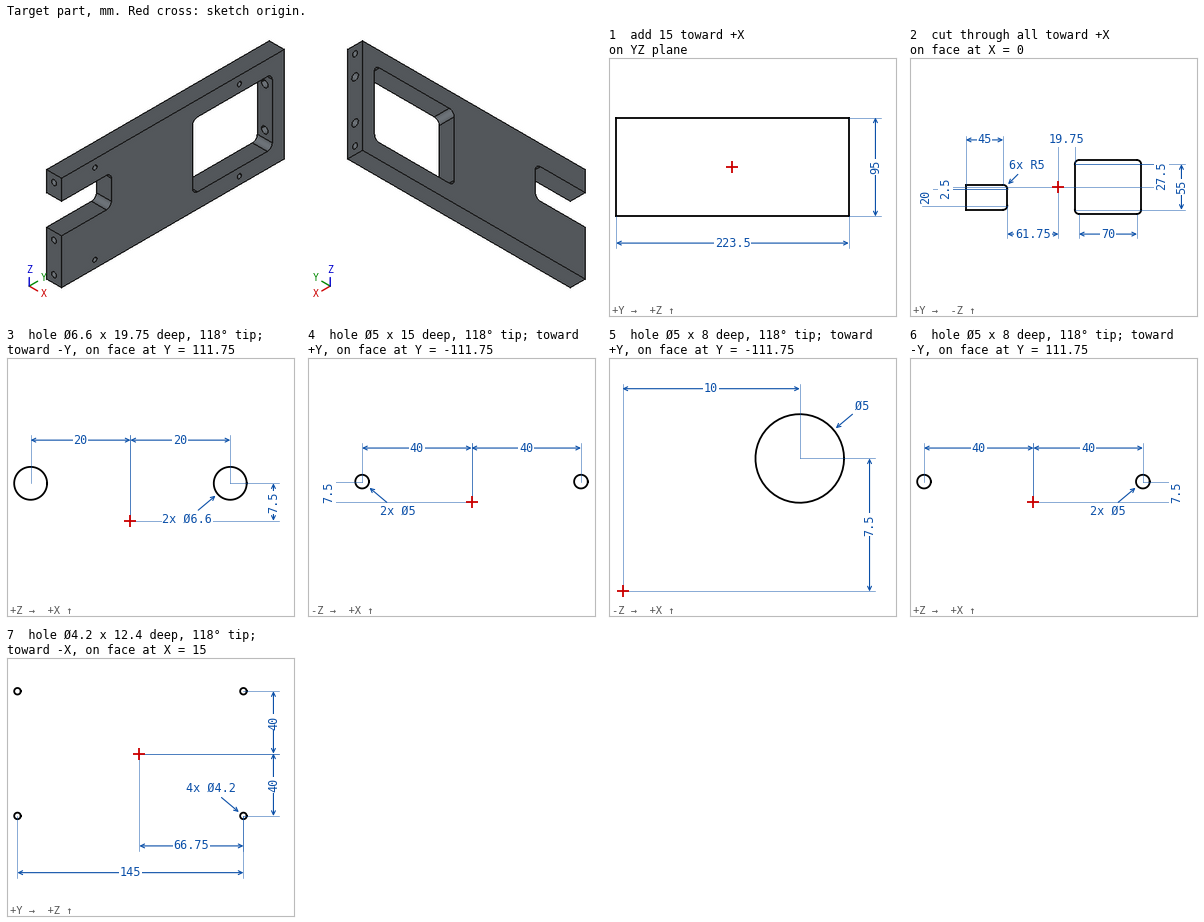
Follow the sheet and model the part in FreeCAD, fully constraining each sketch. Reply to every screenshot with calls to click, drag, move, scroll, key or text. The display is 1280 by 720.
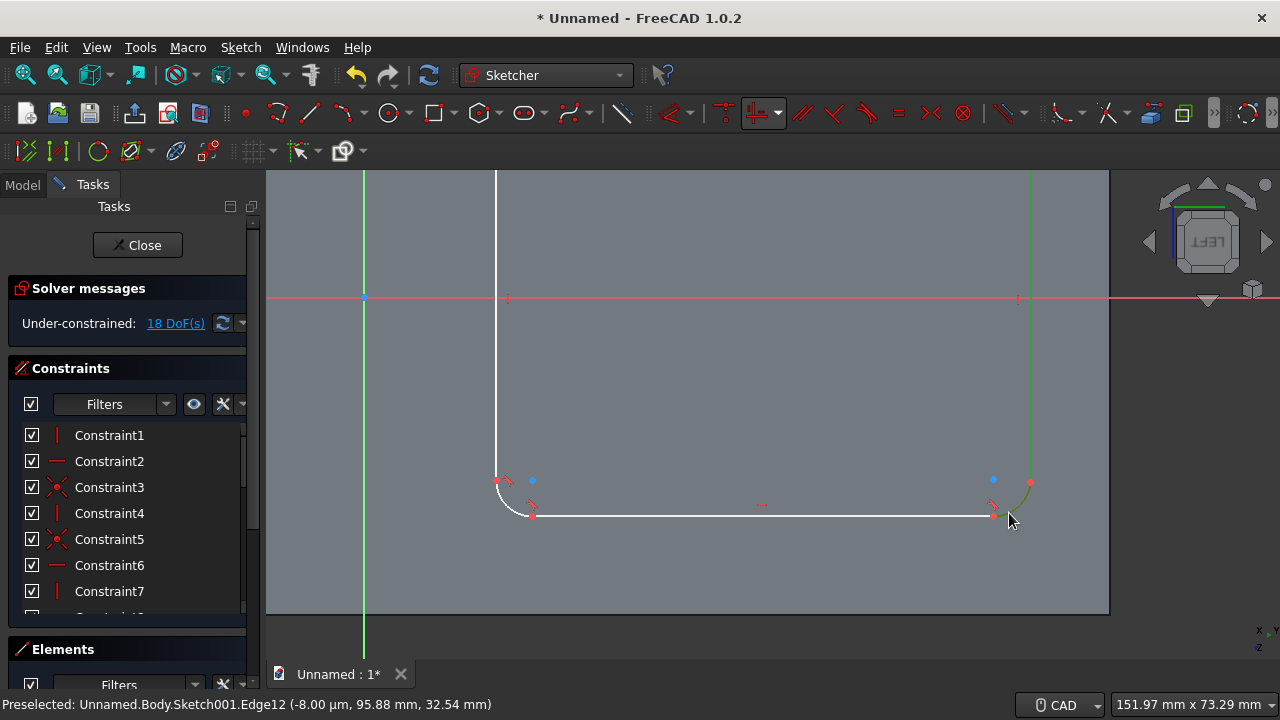
click(868, 114)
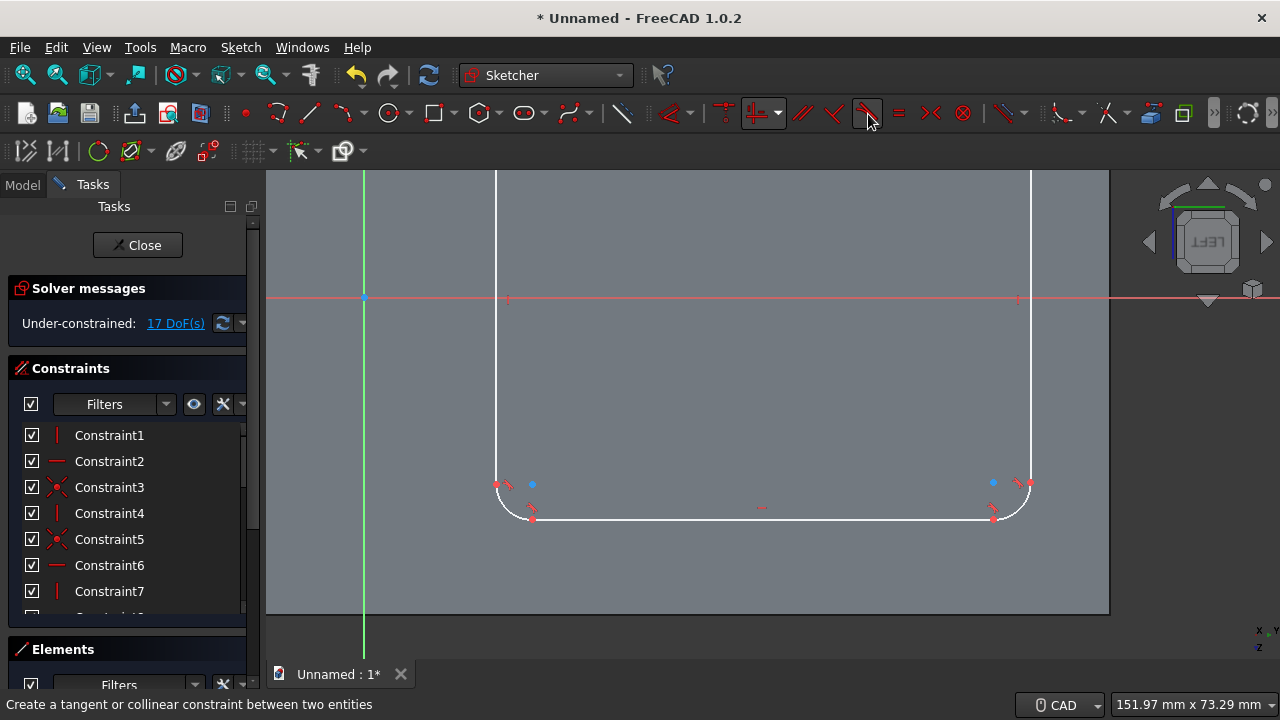
click(1031, 373)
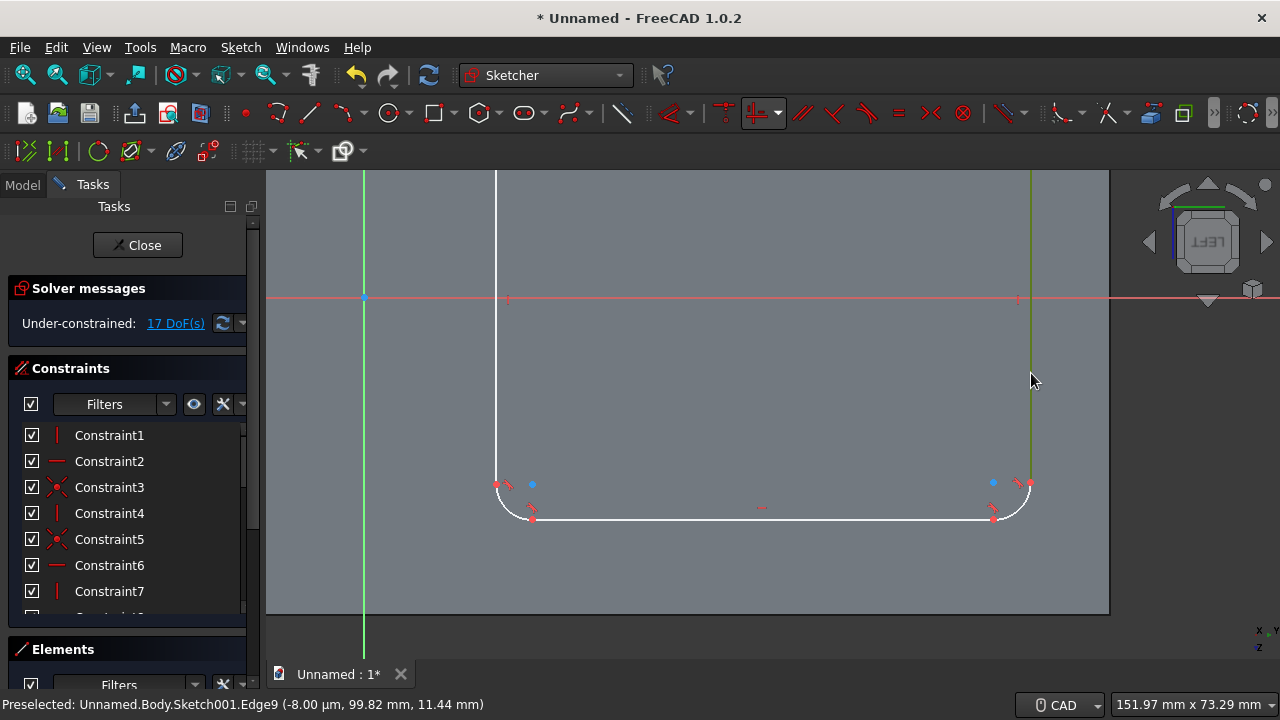
scroll(1015, 510, down, 4)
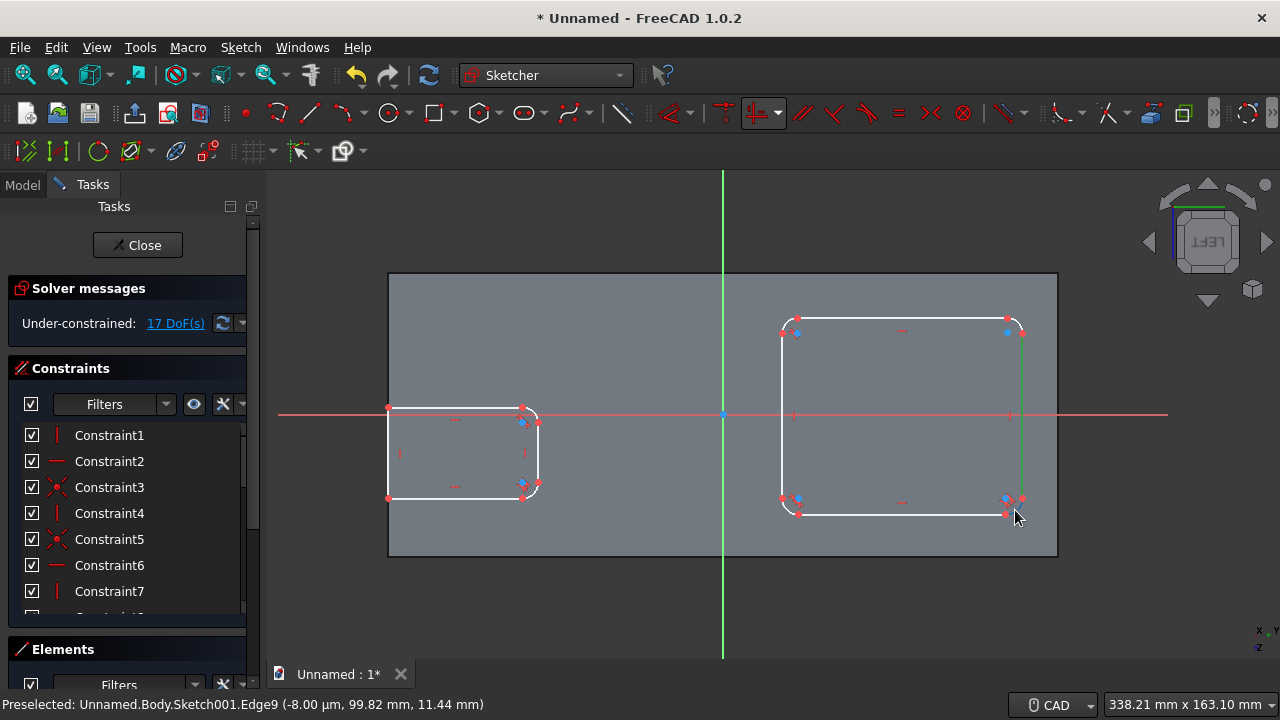
scroll(1021, 326, up, 4)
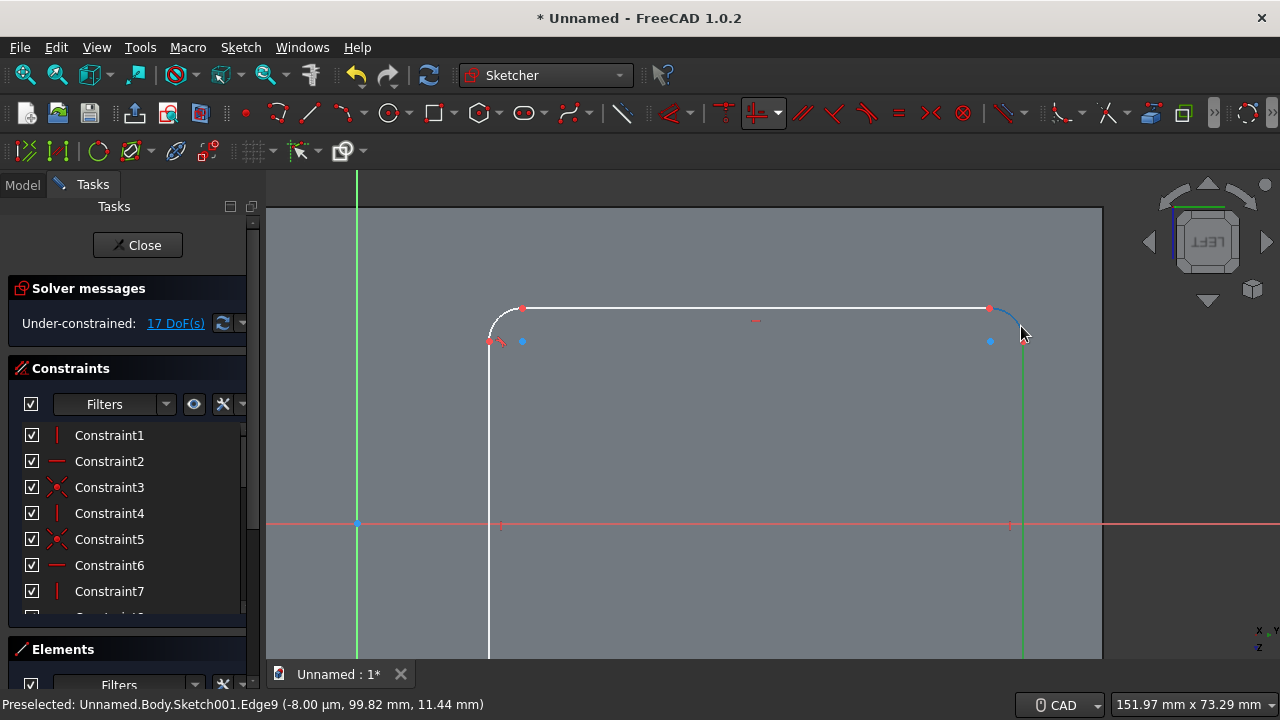
click(1020, 326)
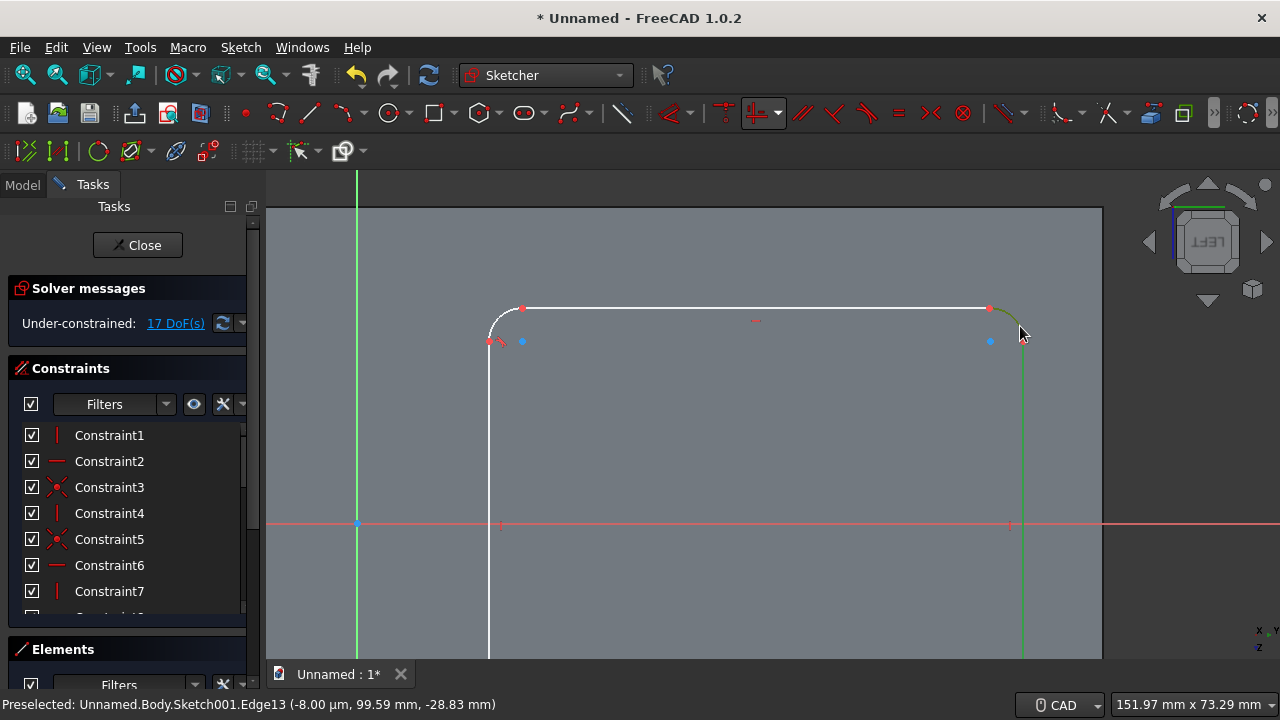
click(868, 114)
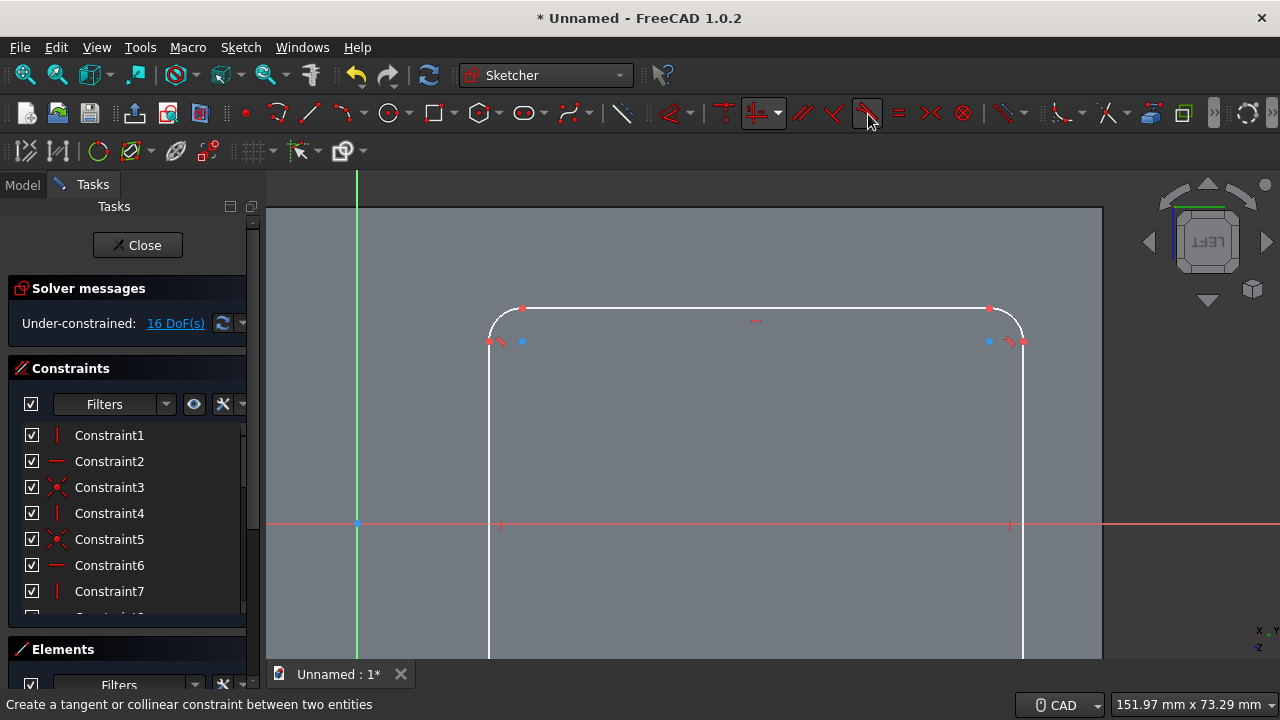
click(850, 308)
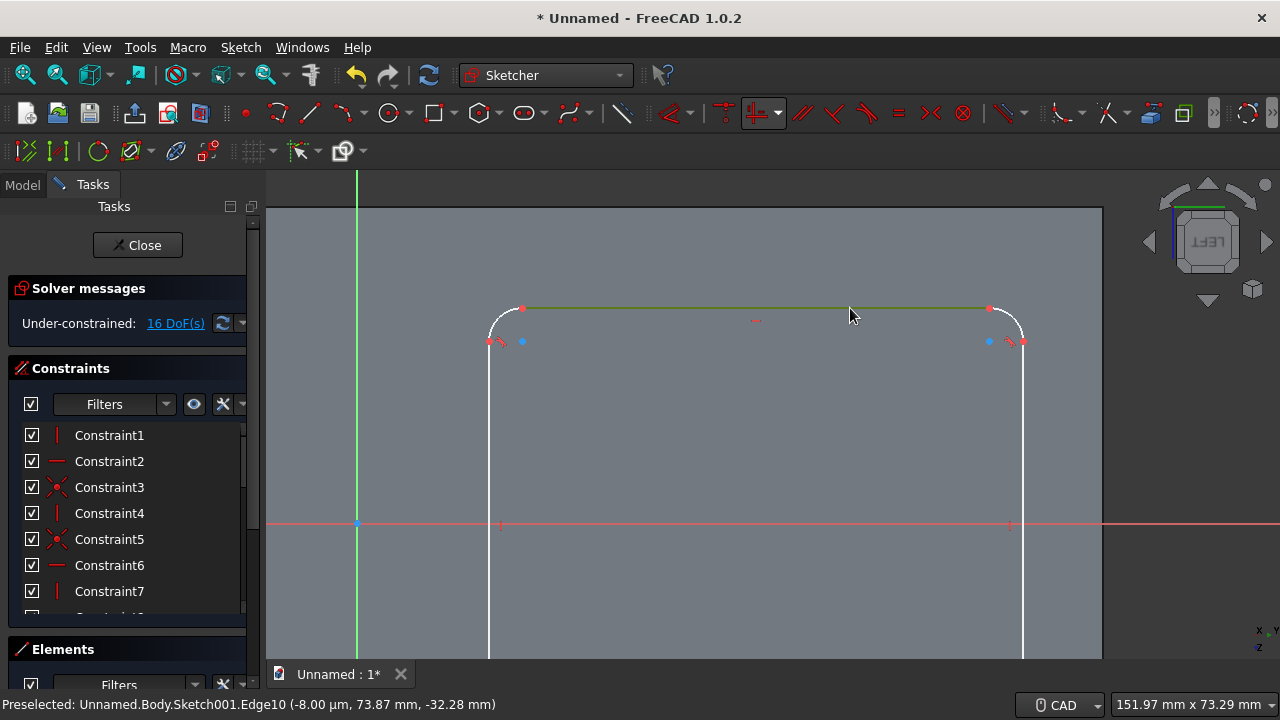
click(1020, 326)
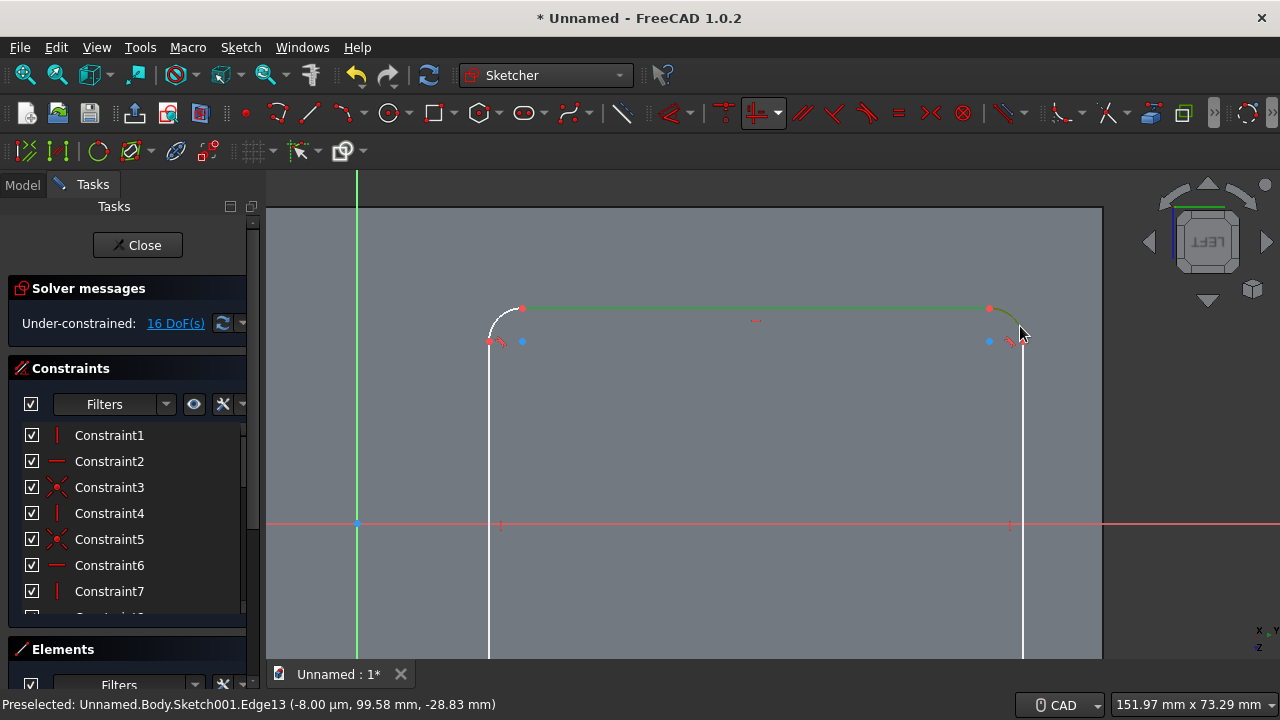
click(868, 114)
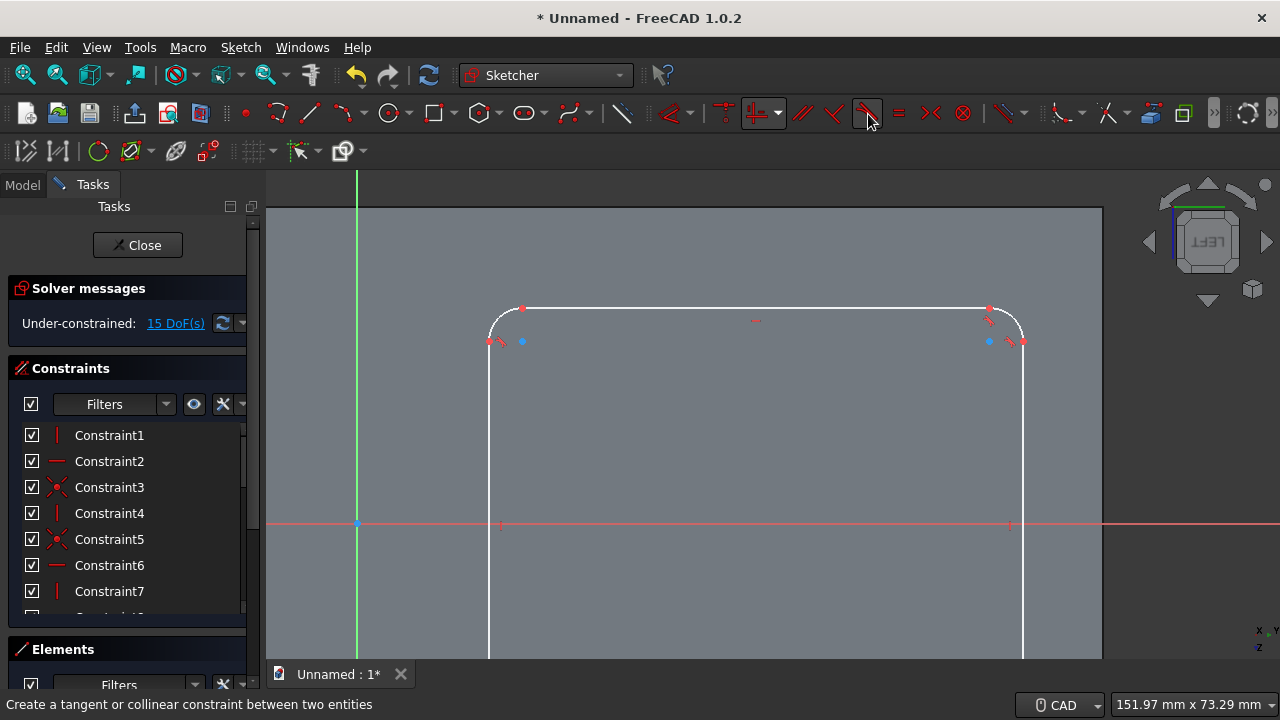
click(850, 308)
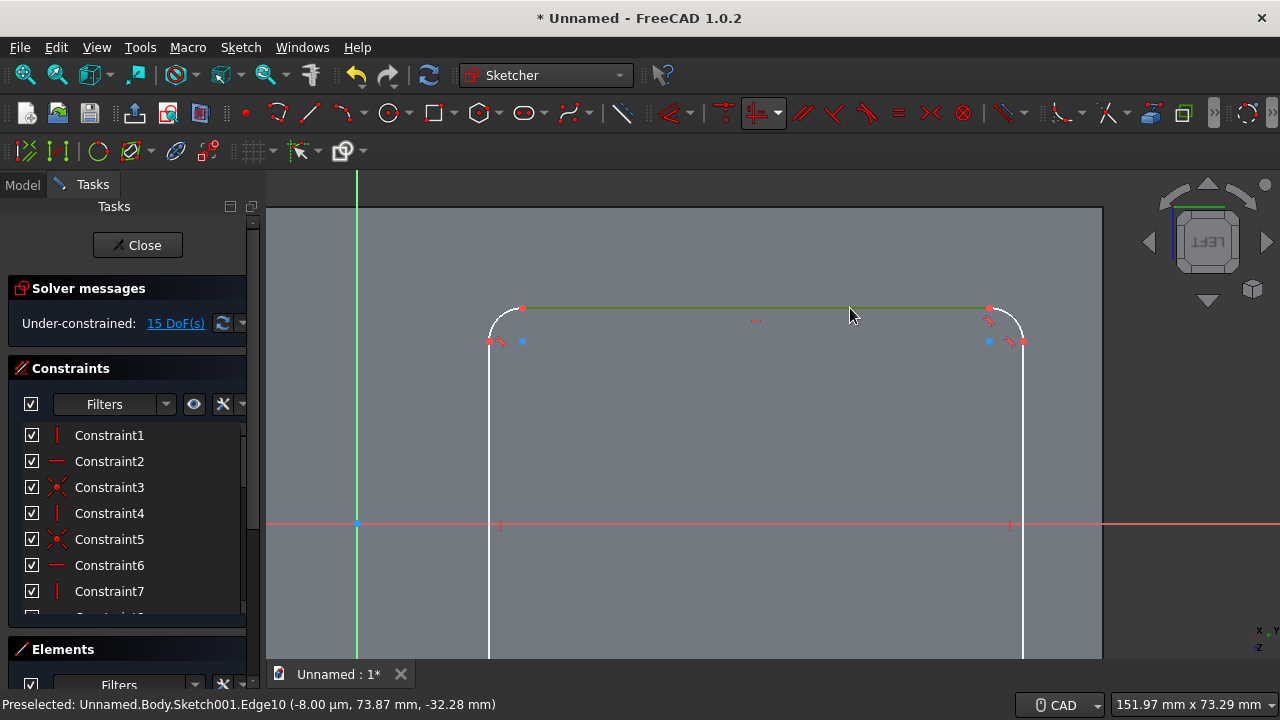
click(507, 312)